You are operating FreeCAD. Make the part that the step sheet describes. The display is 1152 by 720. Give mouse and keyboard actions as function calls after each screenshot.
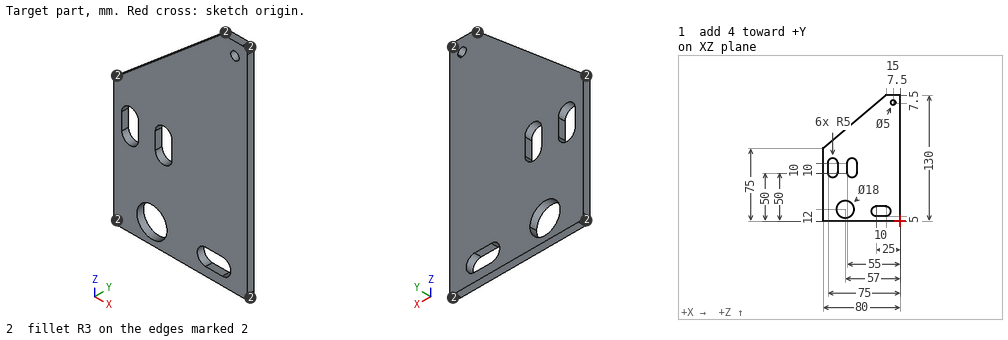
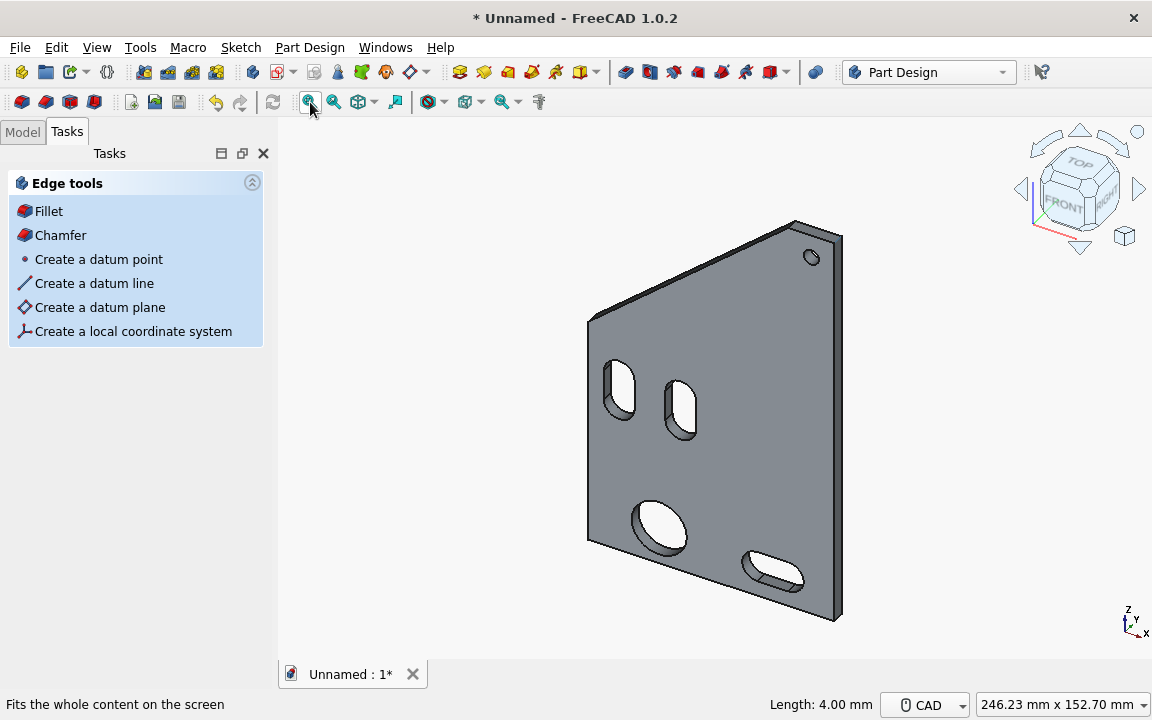
key(0)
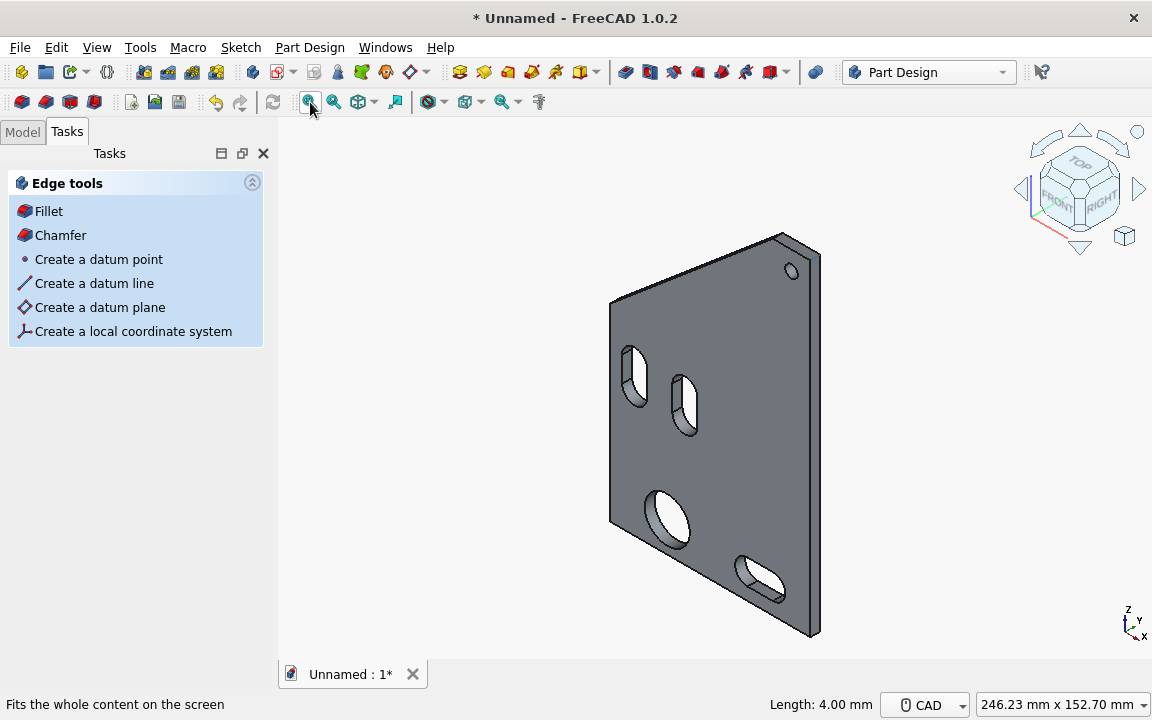
scroll(778, 235, up, 6)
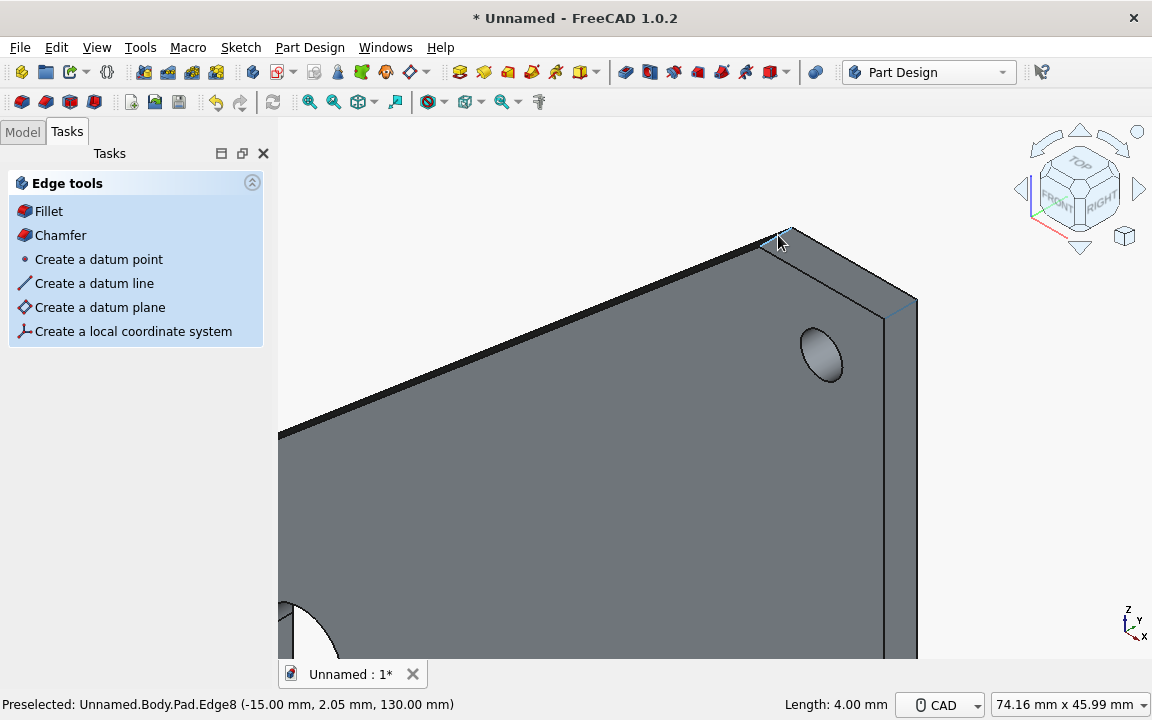
key(v)
key(f)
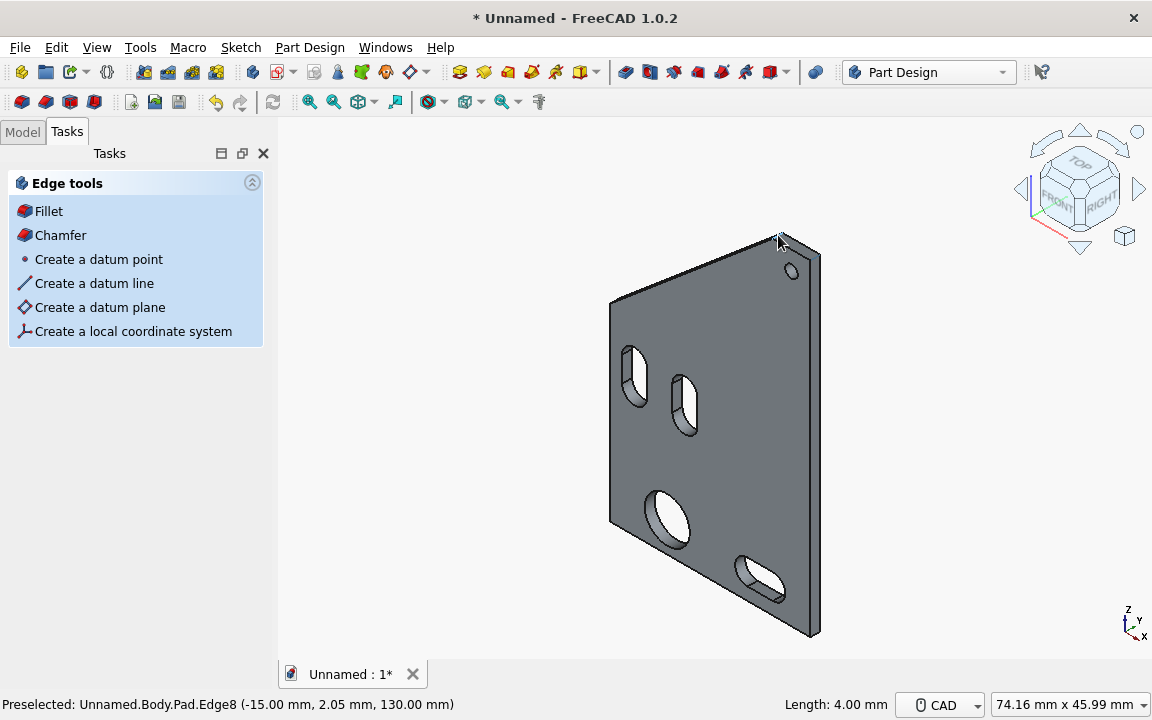
key(2)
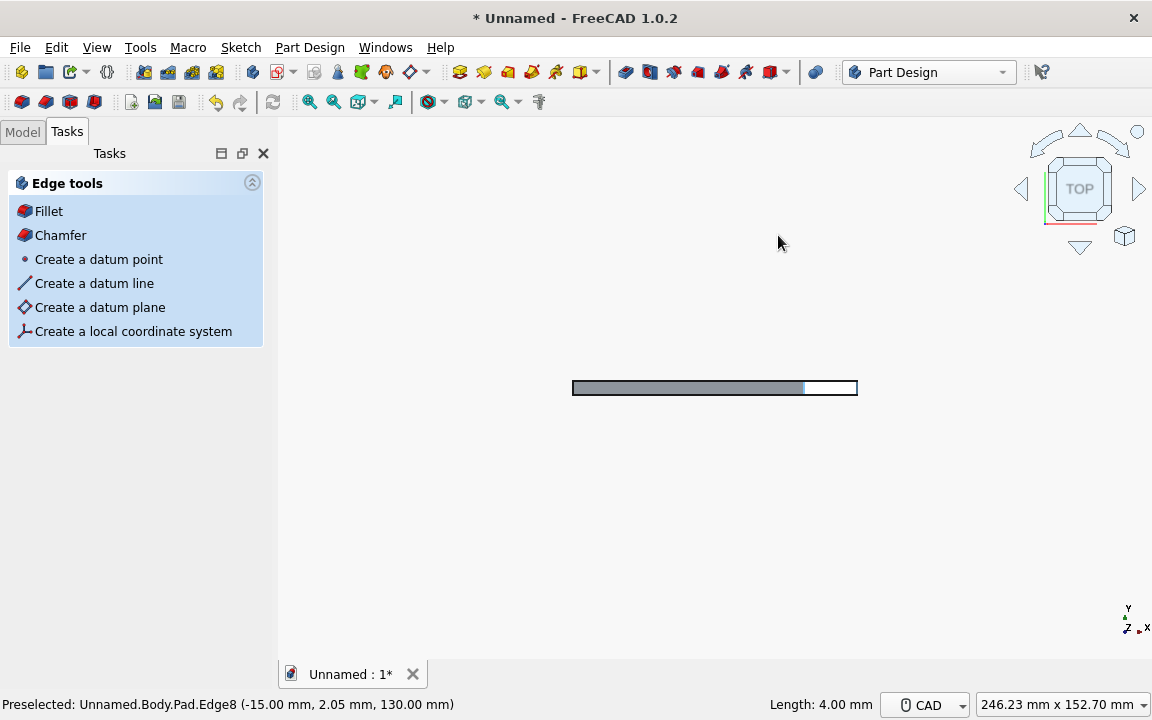
click(310, 102)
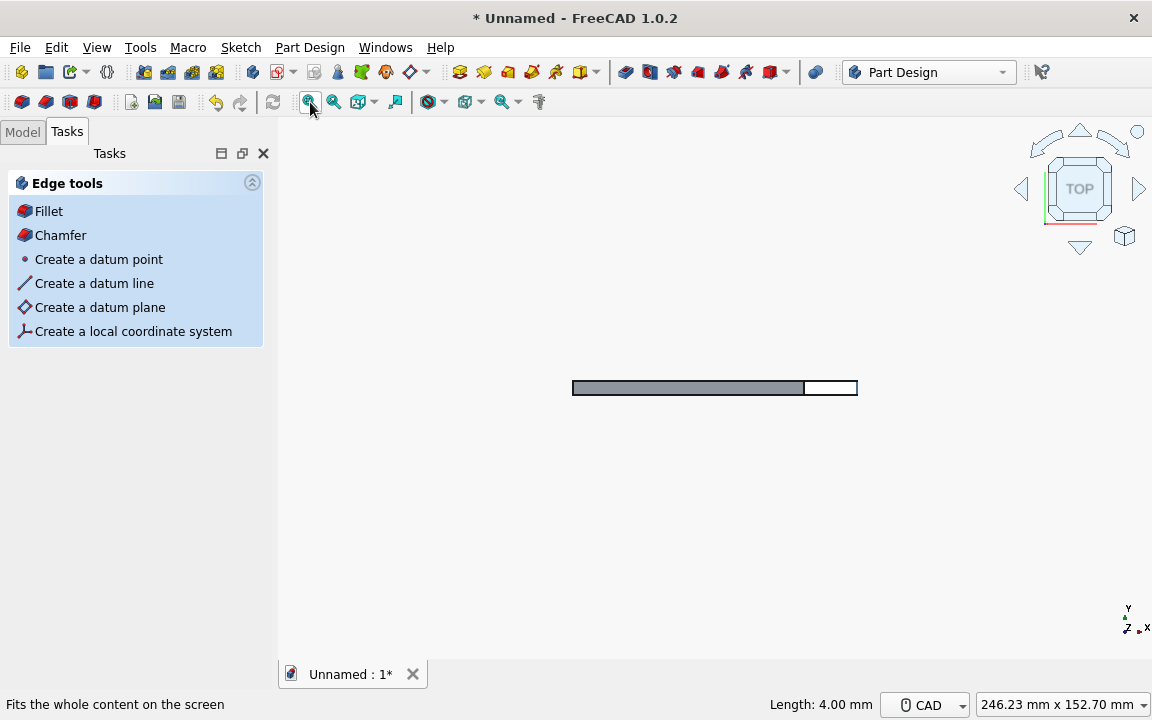
click(804, 387, ctrl)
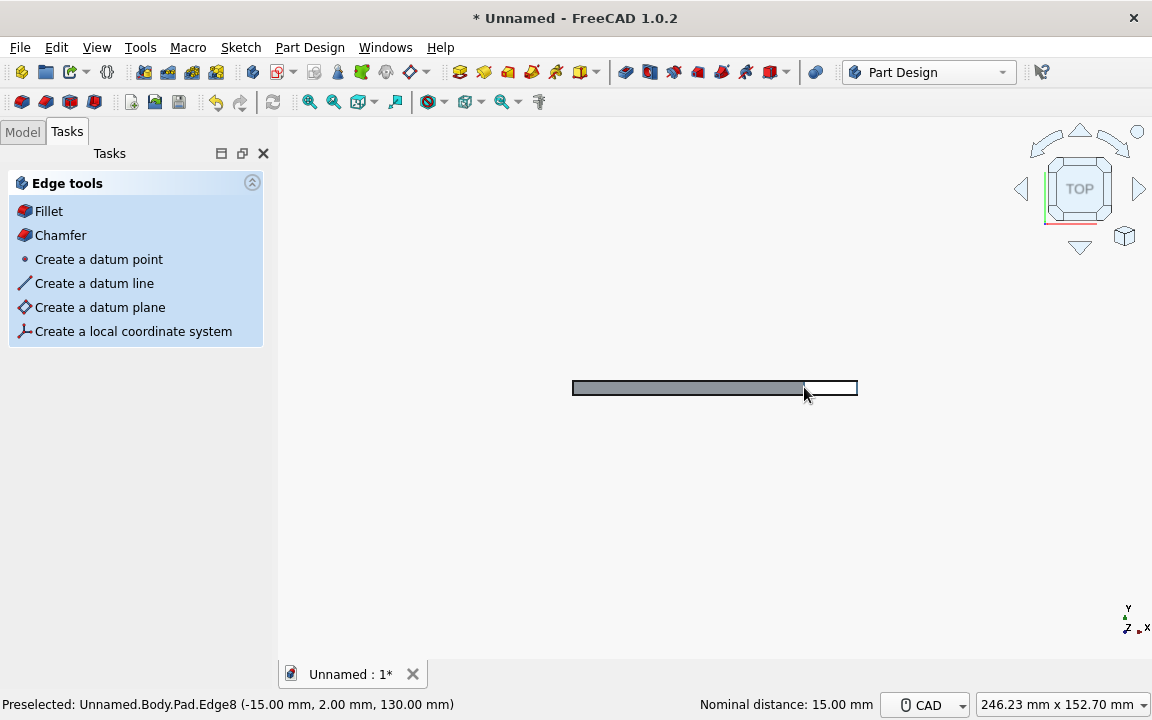
scroll(573, 387, up, 6)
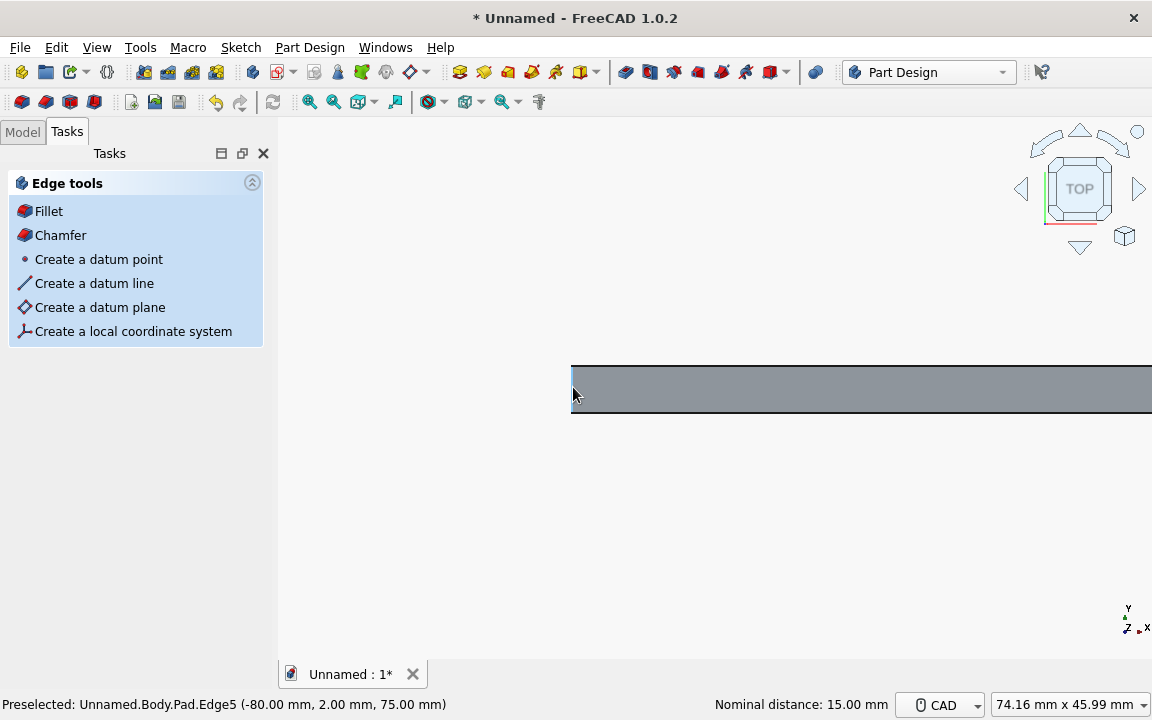
click(310, 102)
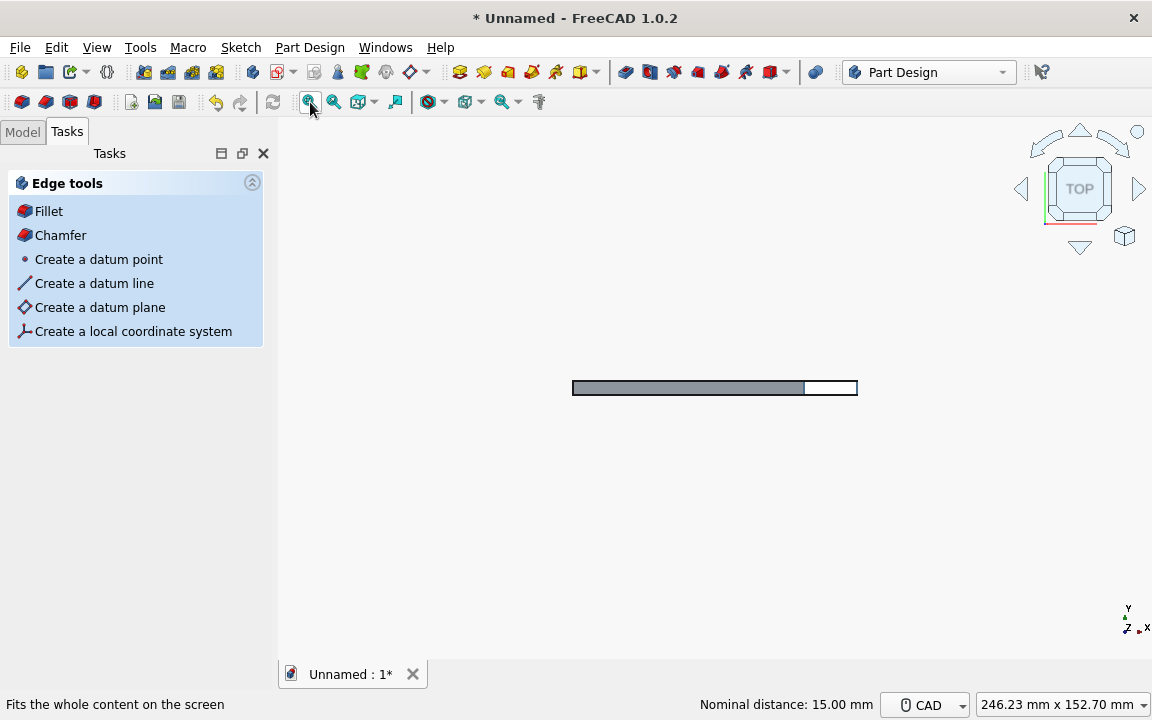
key(1)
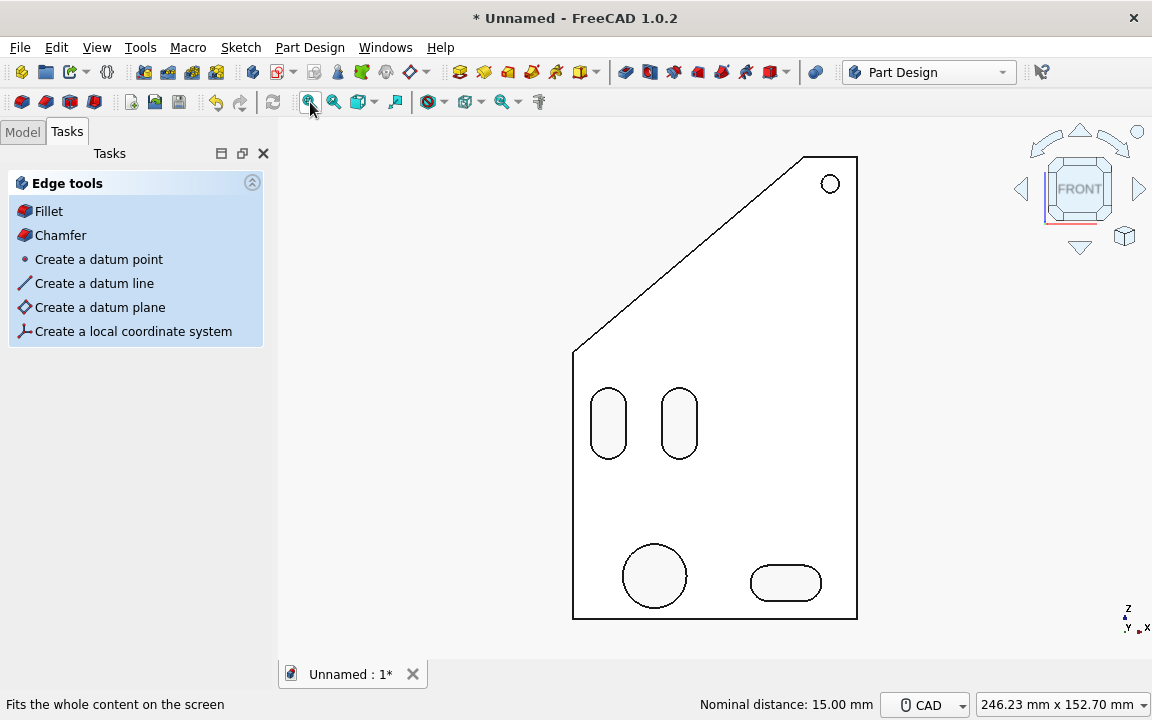
scroll(573, 352, up, 6)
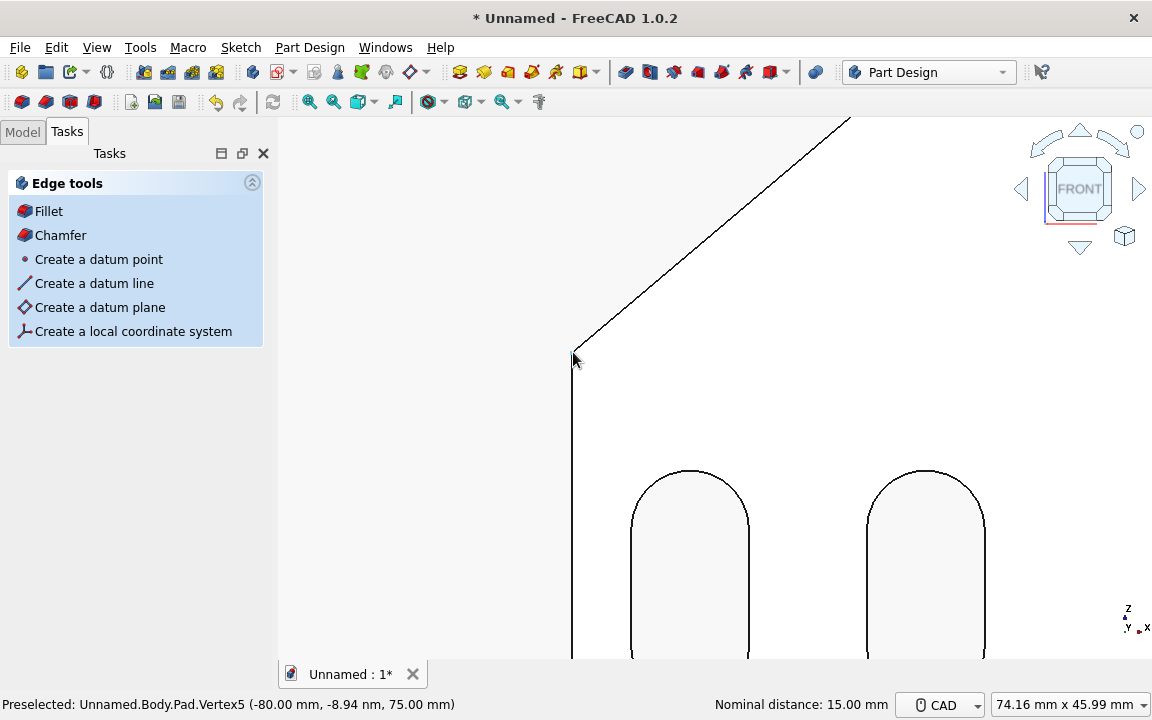
key(v)
key(f)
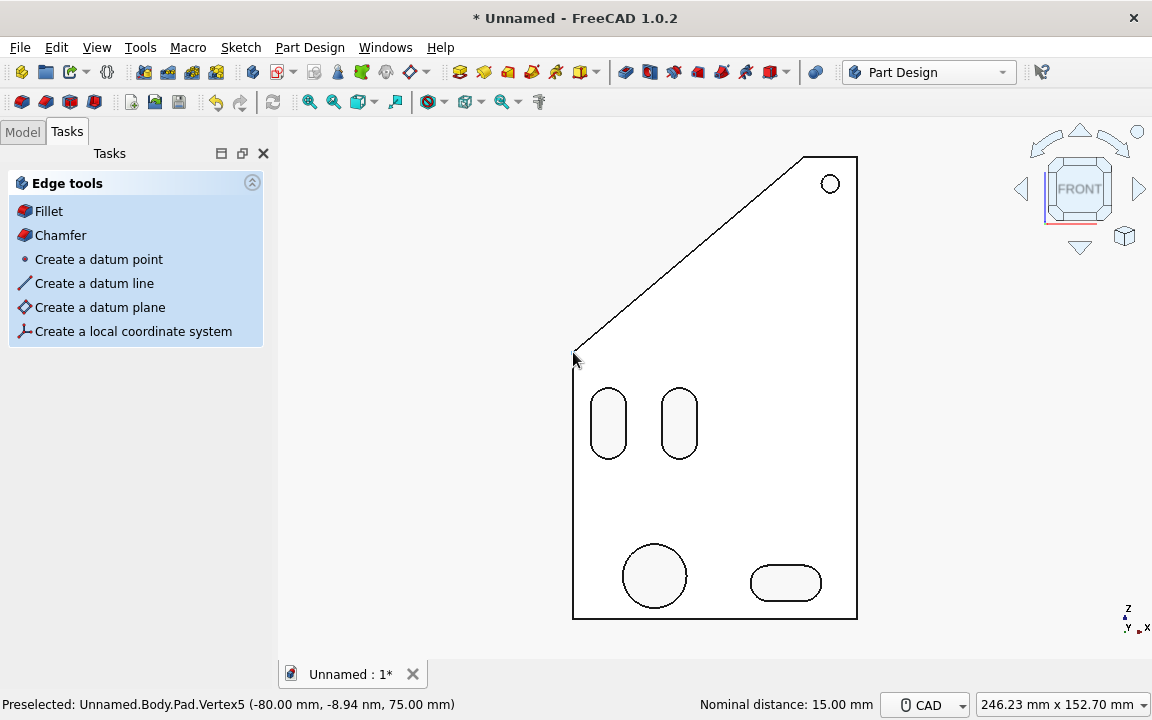
key(3)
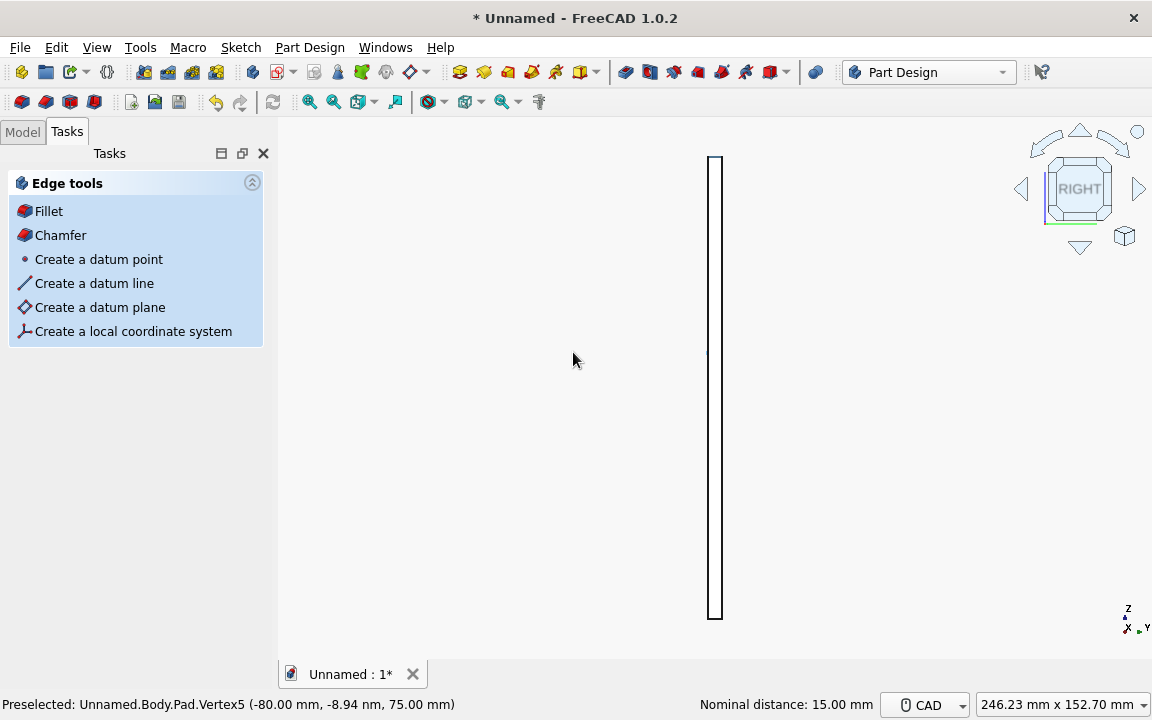
click(715, 618, ctrl)